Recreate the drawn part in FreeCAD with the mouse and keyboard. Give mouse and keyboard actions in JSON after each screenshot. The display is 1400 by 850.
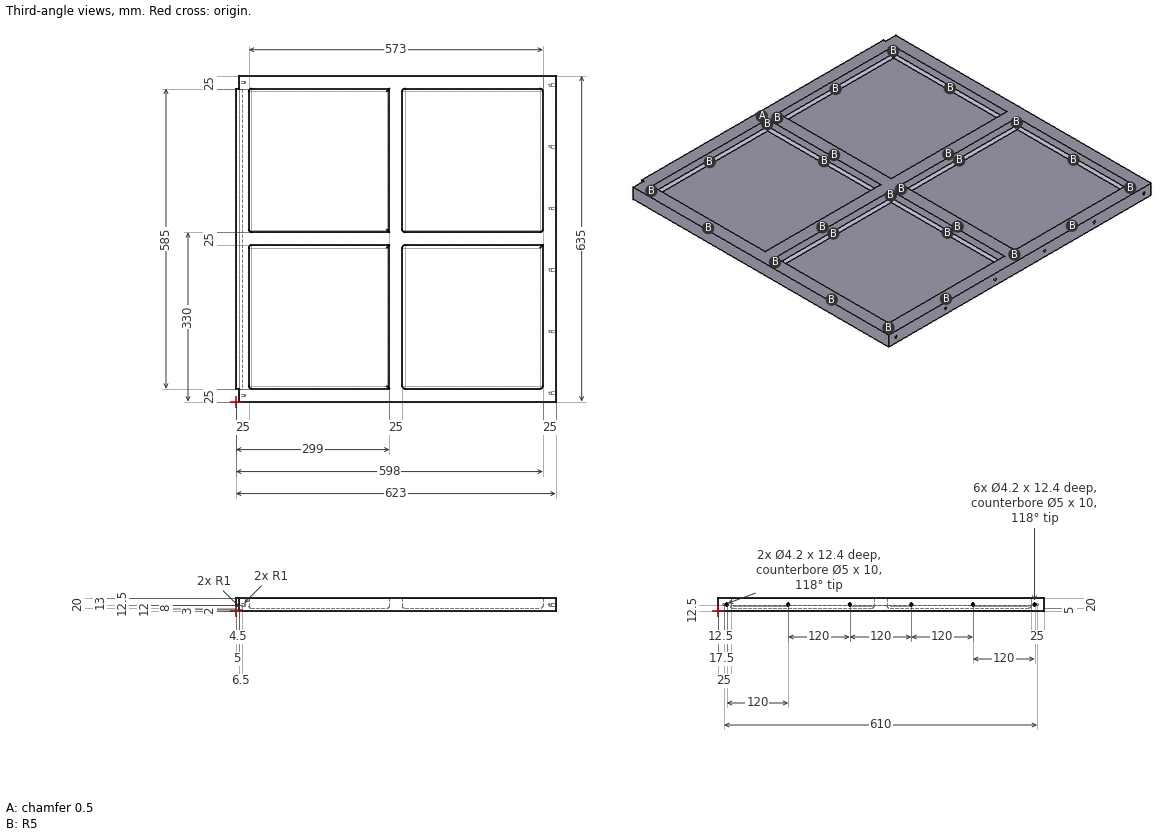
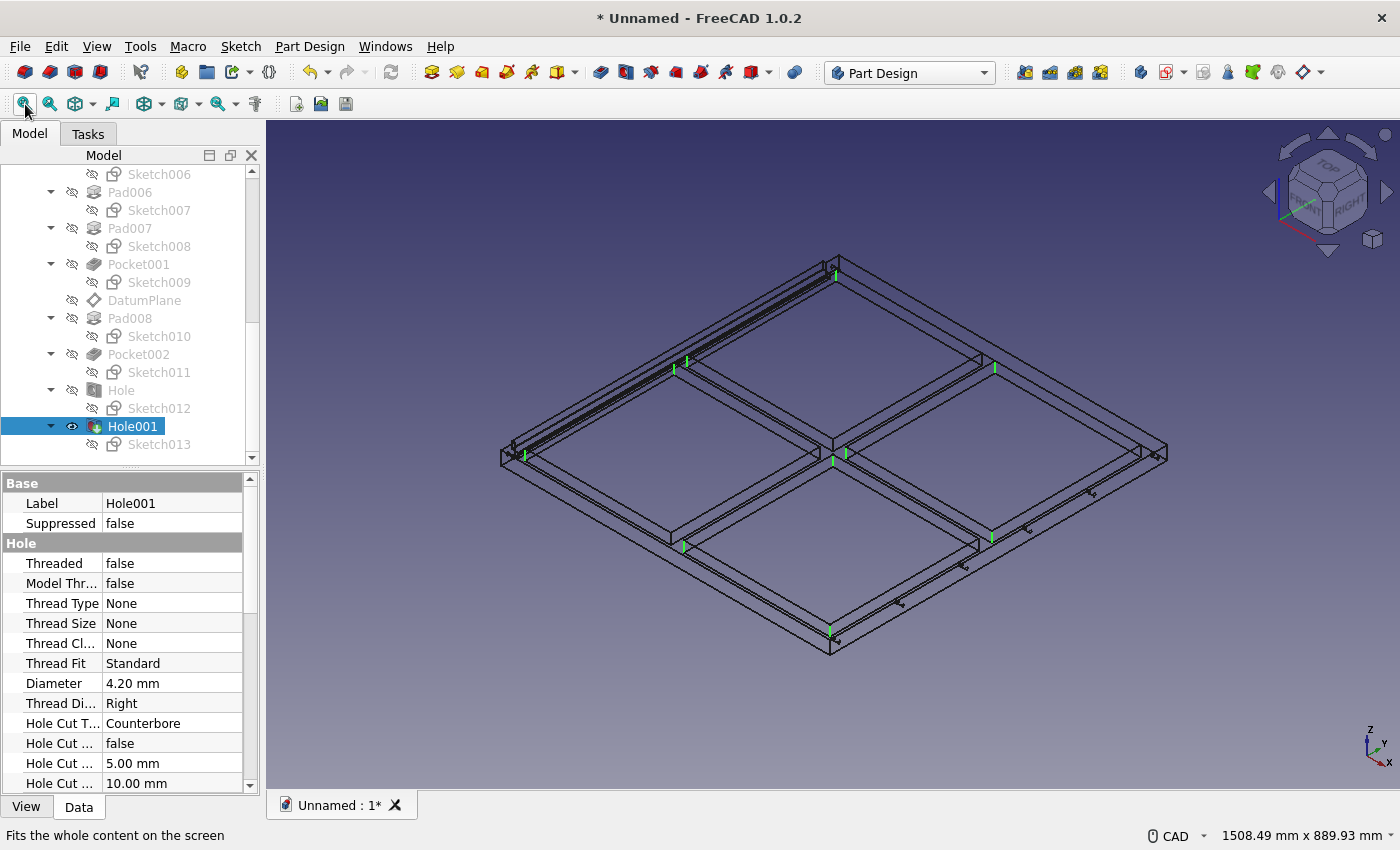
{"action": "key", "text": "2"}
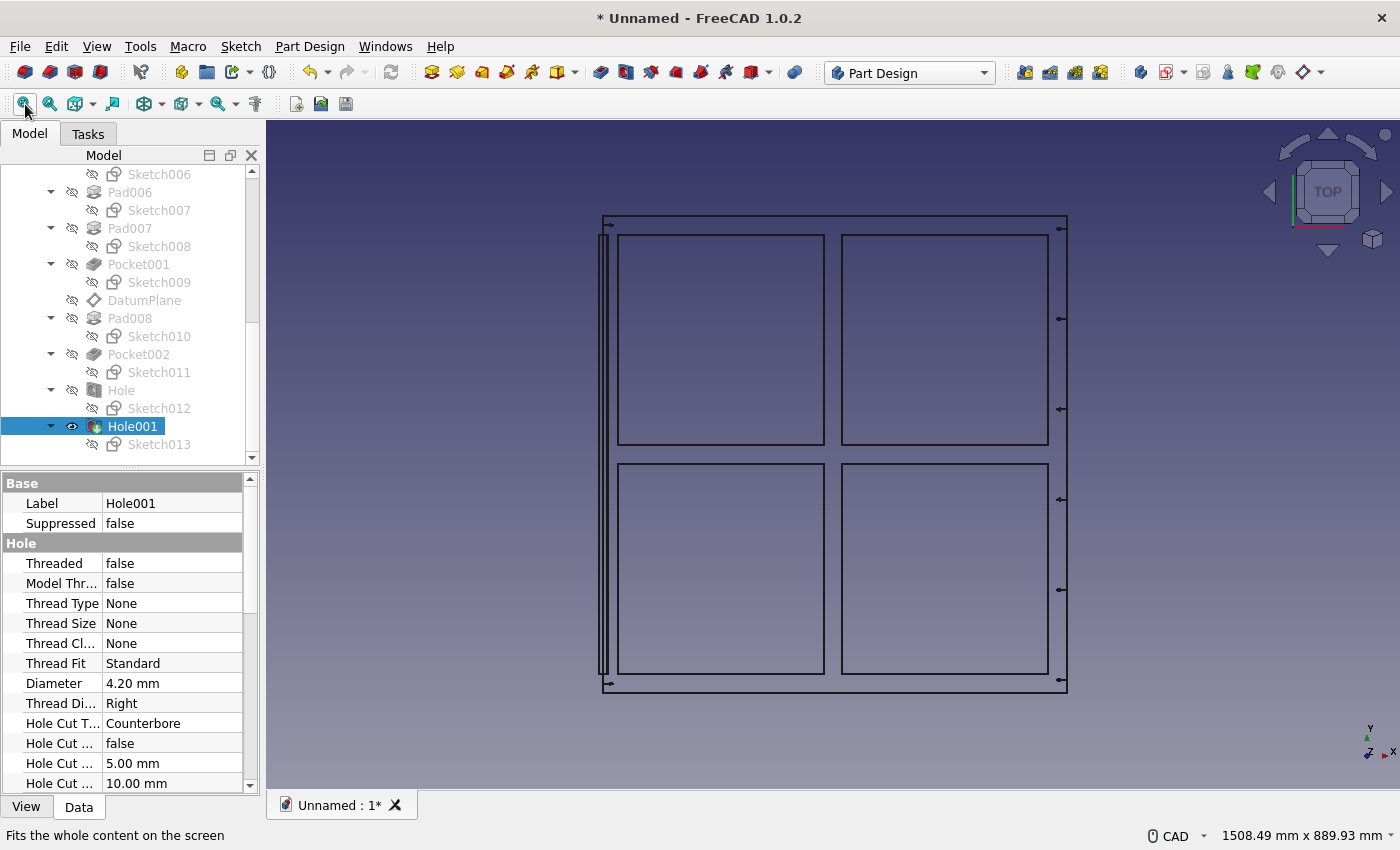
{"action": "scroll", "coordinate": [1048, 234], "scroll_direction": "up", "scroll_amount": 6}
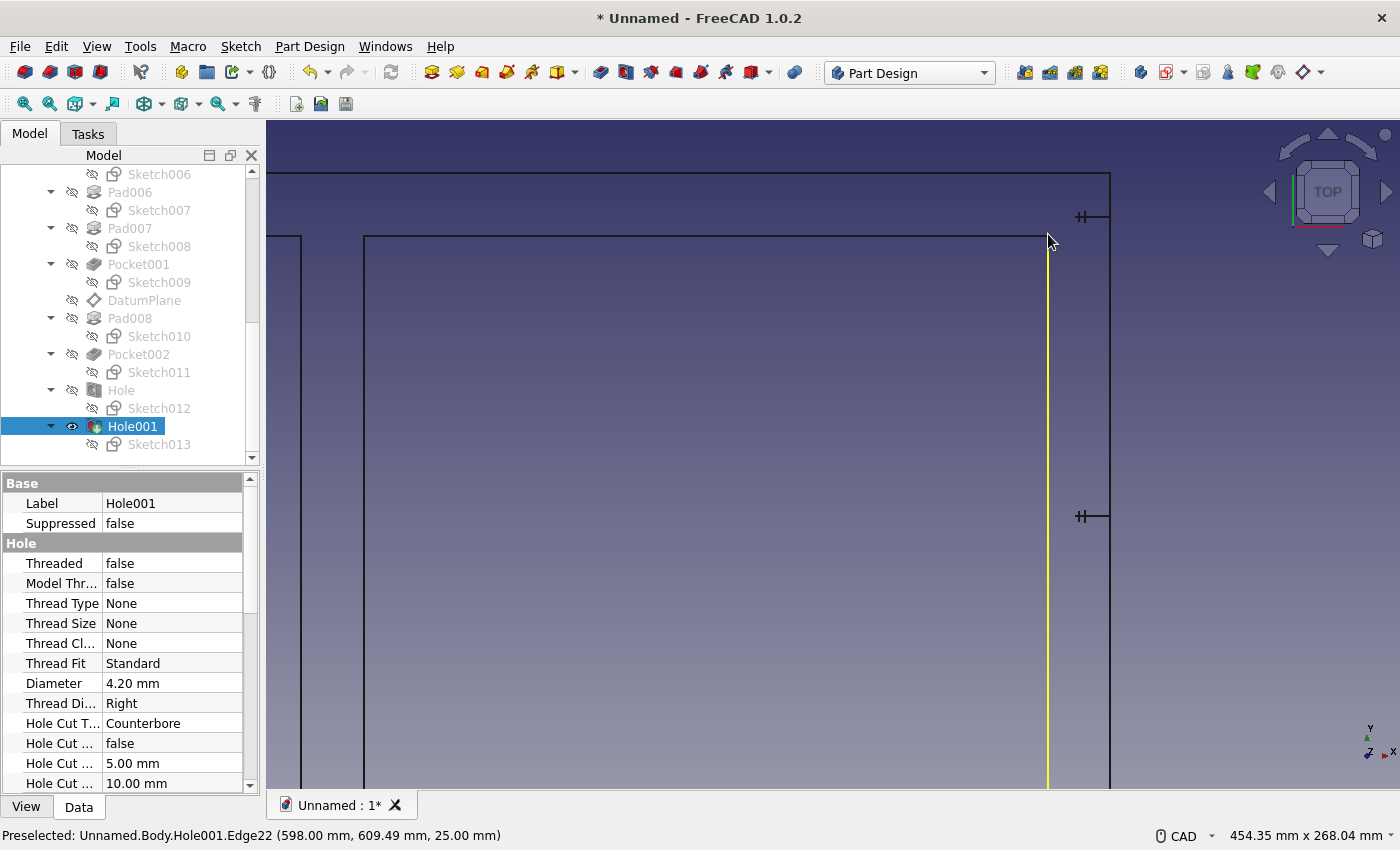
{"action": "left_click", "coordinate": [25, 104]}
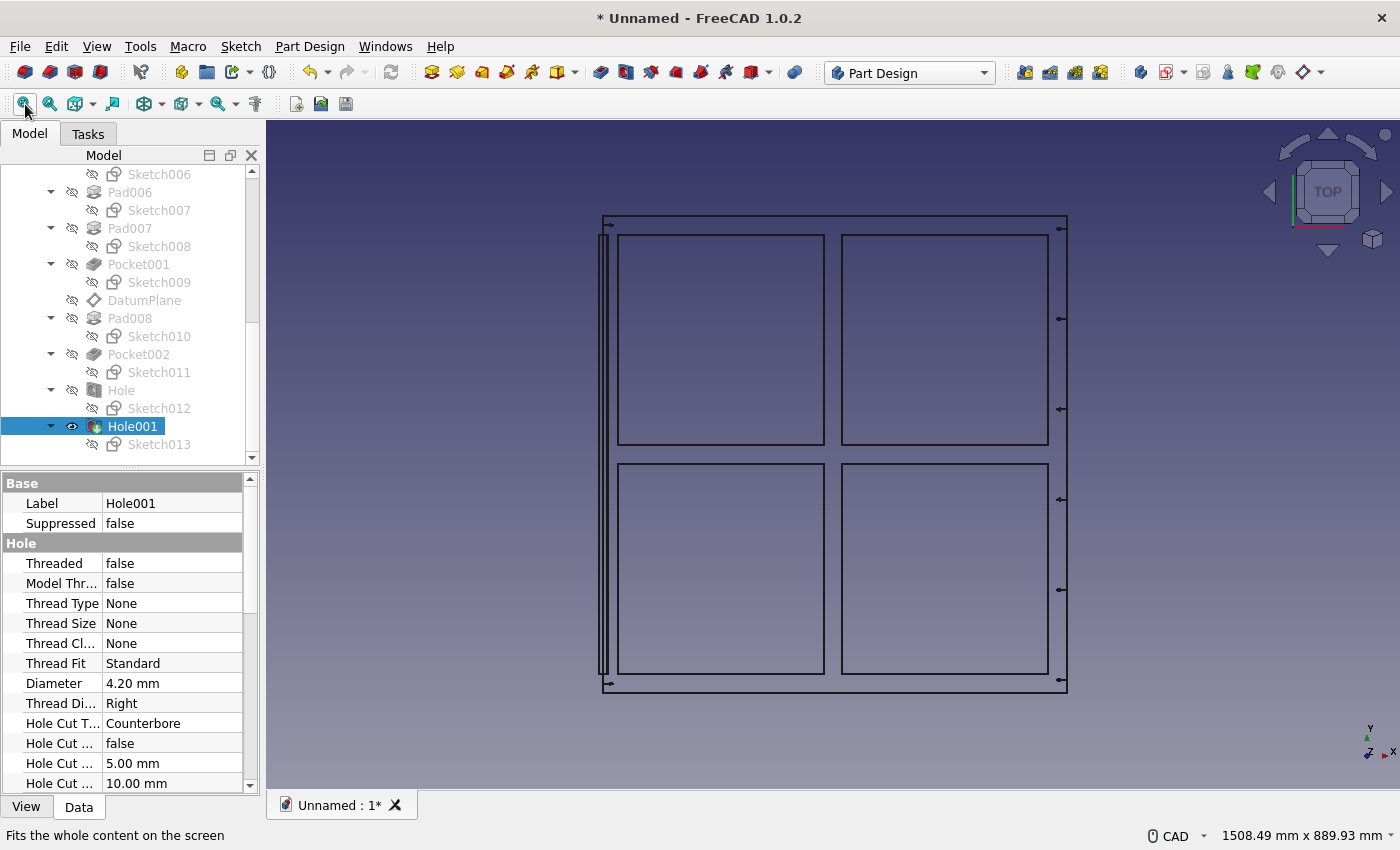
{"action": "key", "text": "1"}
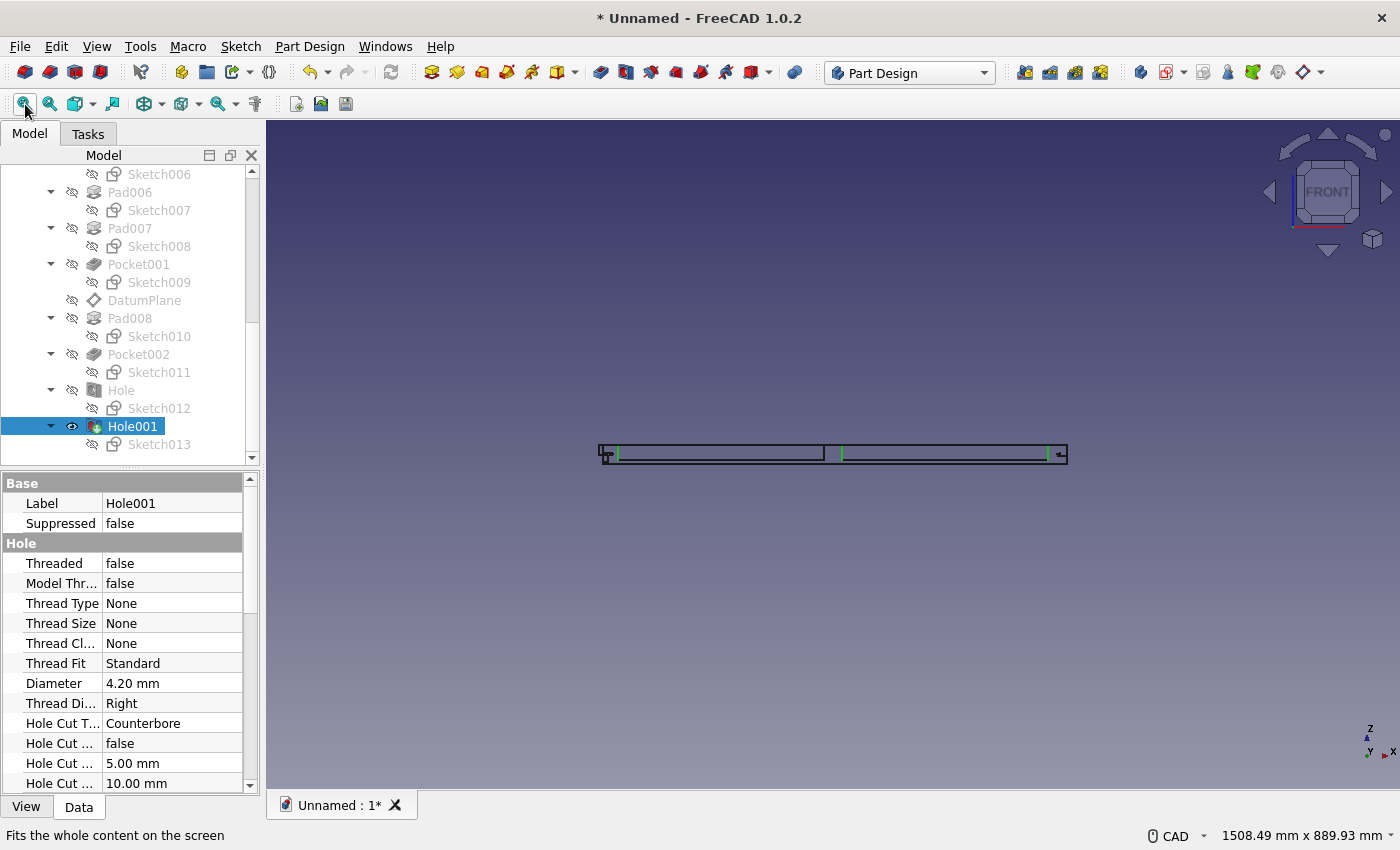
{"action": "left_click", "coordinate": [25, 104]}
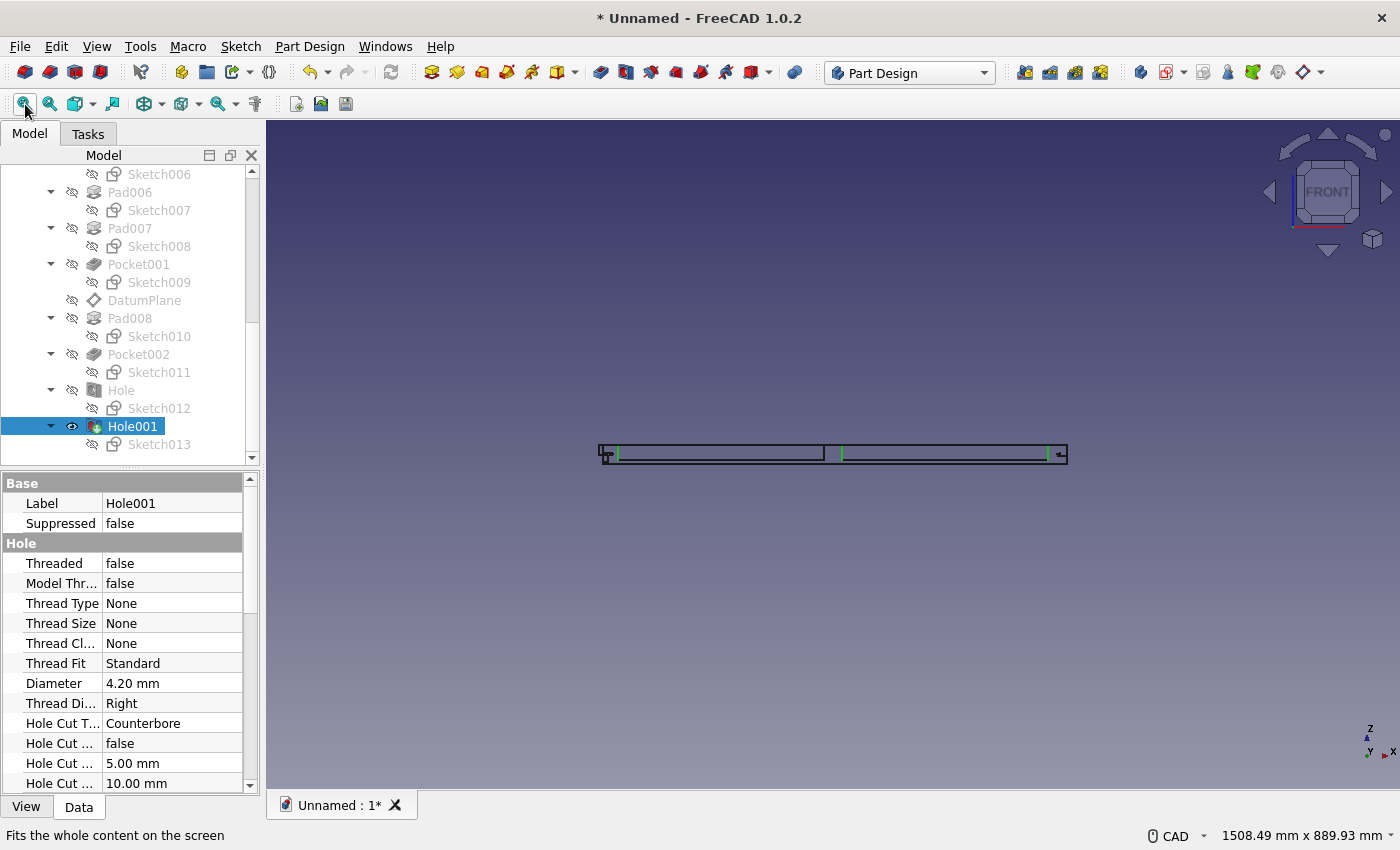
{"action": "scroll", "coordinate": [1048, 452], "scroll_direction": "up", "scroll_amount": 6}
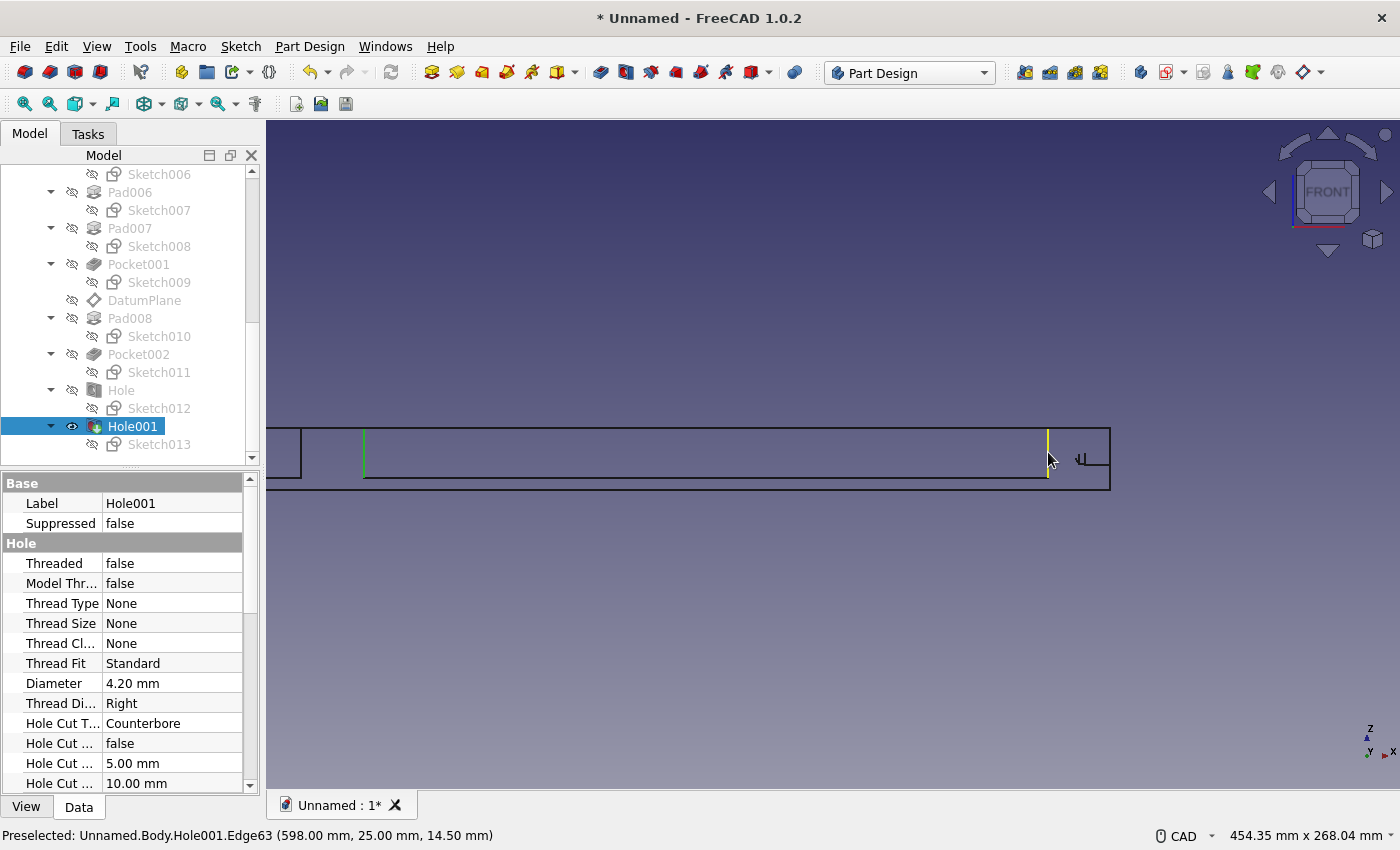
{"action": "left_click", "coordinate": [25, 104]}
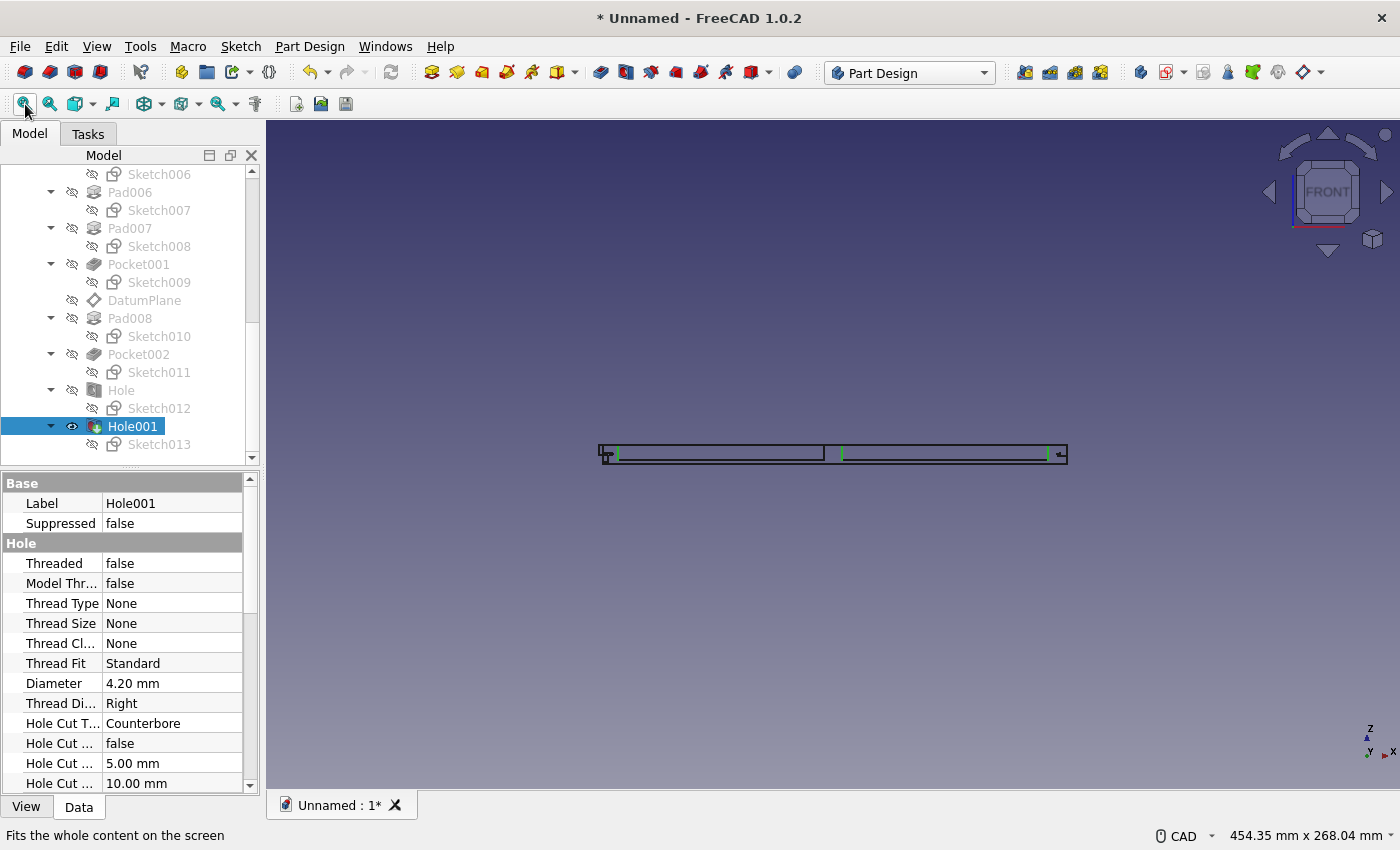
{"action": "key", "text": "3"}